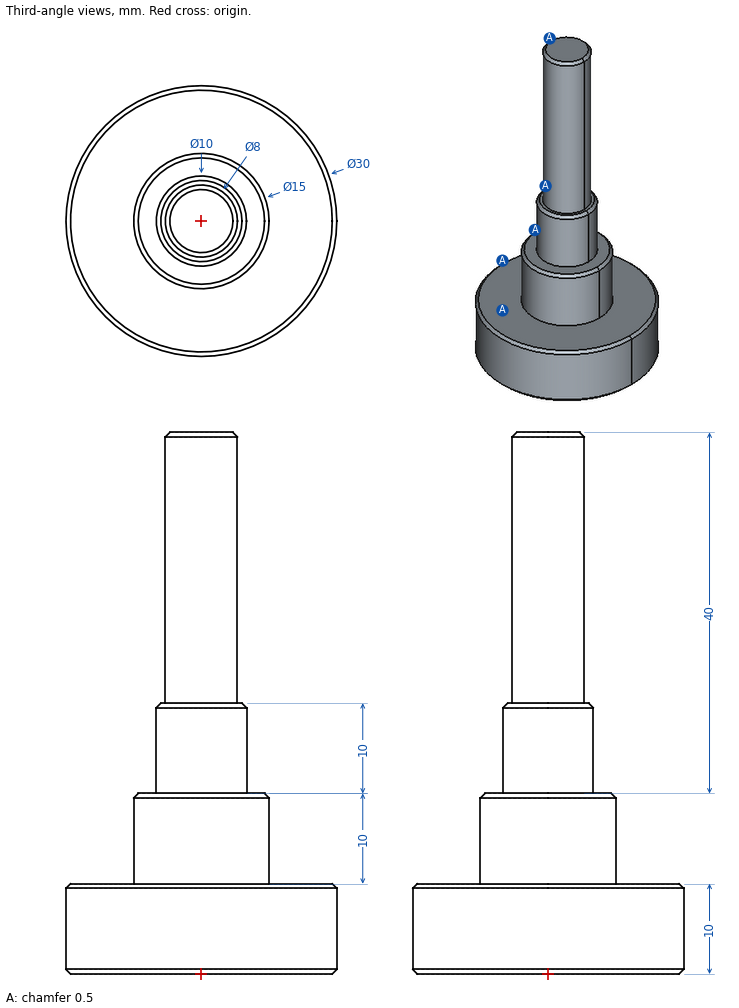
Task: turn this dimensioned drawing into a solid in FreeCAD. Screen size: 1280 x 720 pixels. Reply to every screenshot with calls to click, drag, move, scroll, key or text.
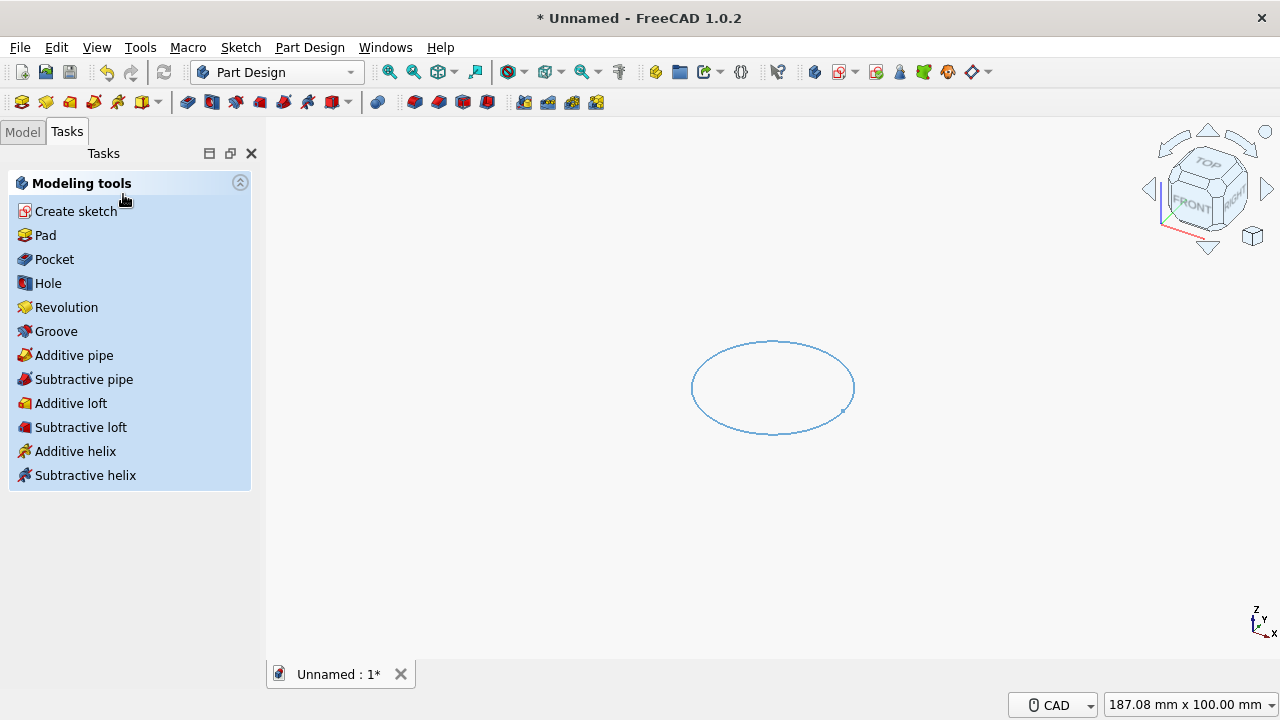
click(22, 102)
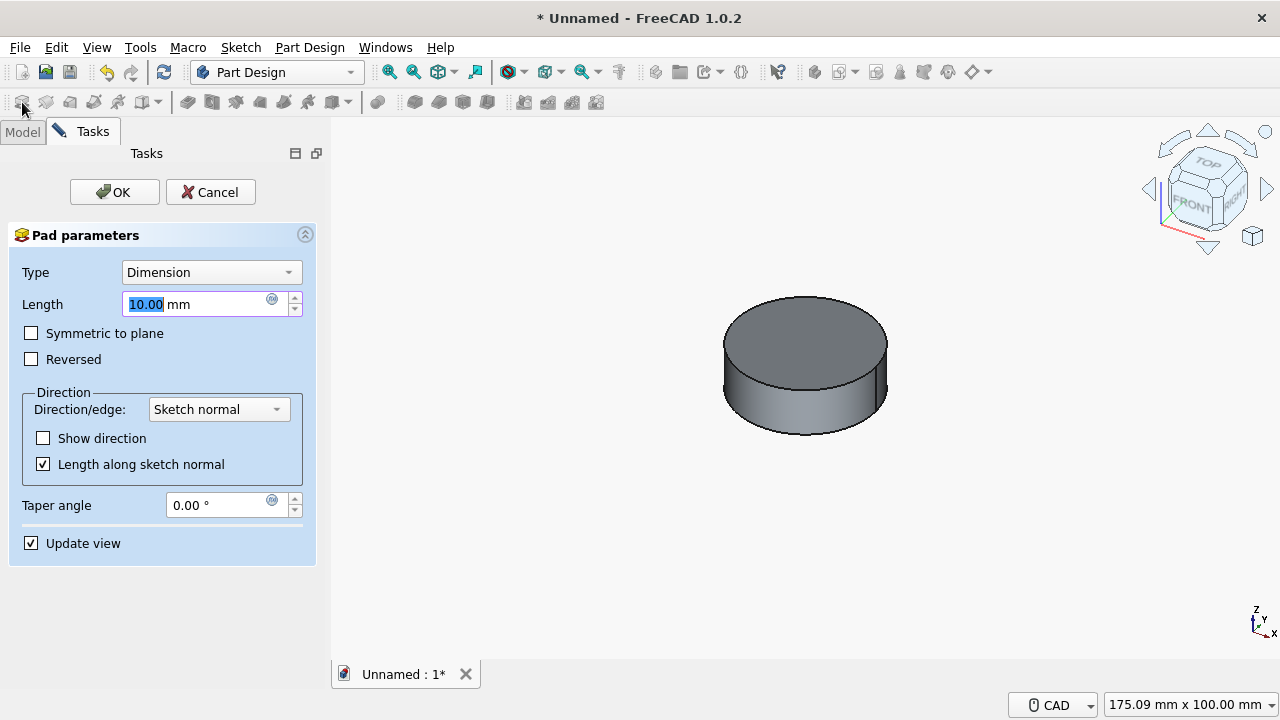
text(10)
key(Tab)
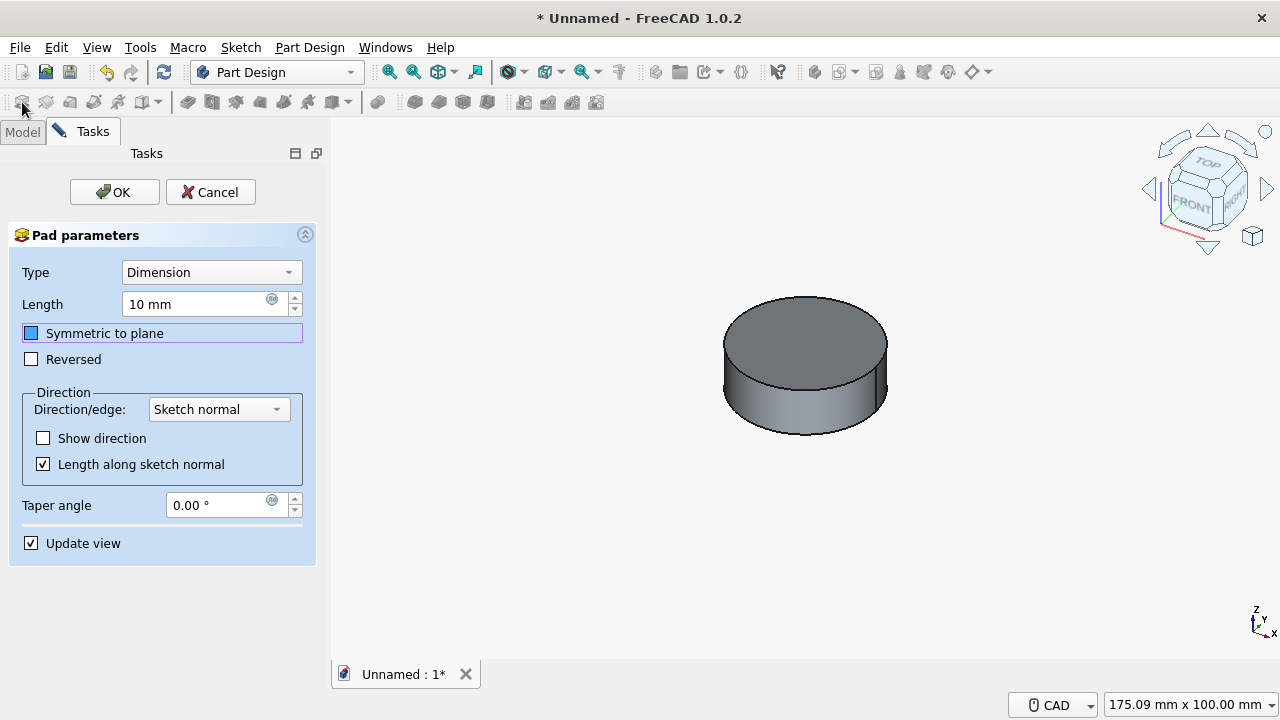
click(115, 192)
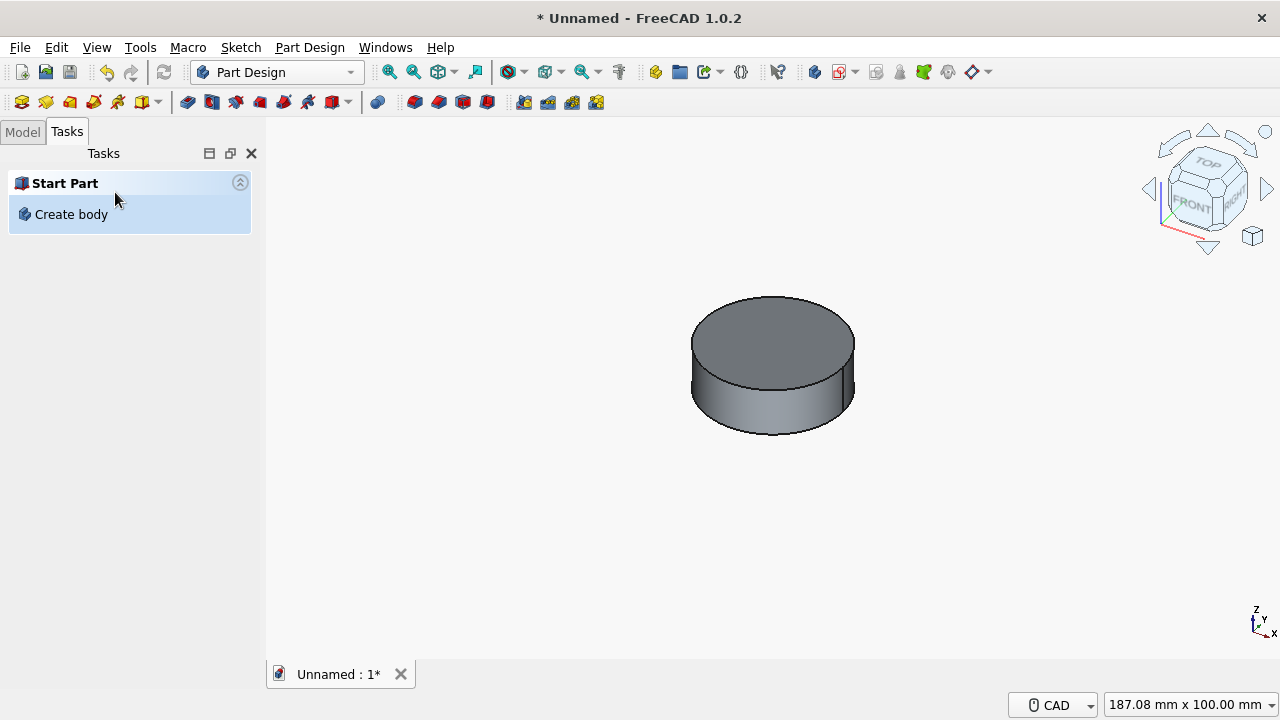
key(v)
key(f)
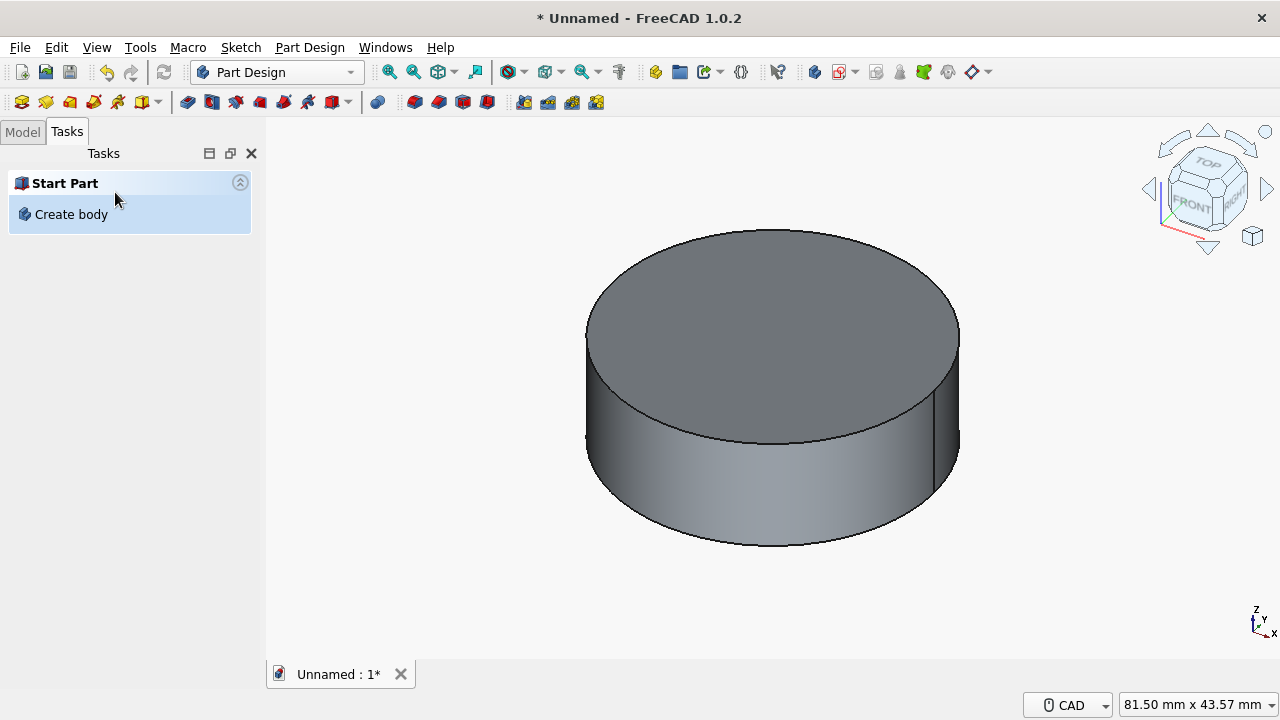
click(773, 336)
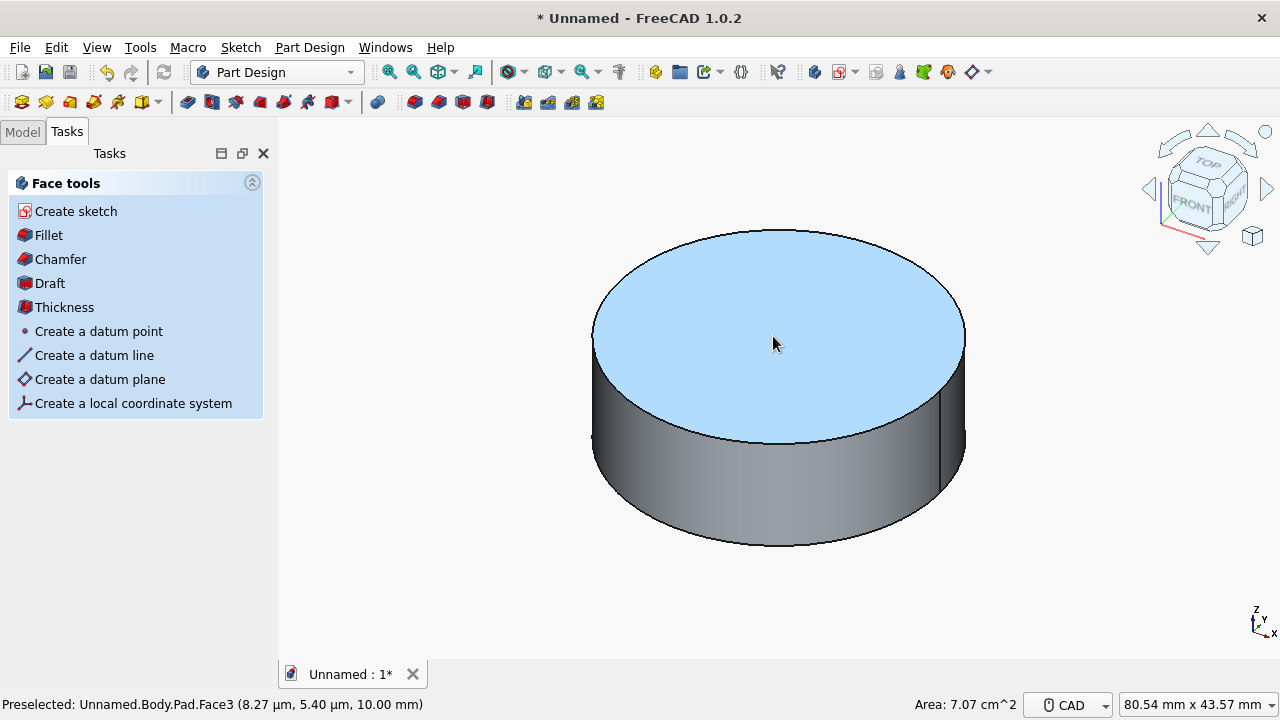
click(840, 72)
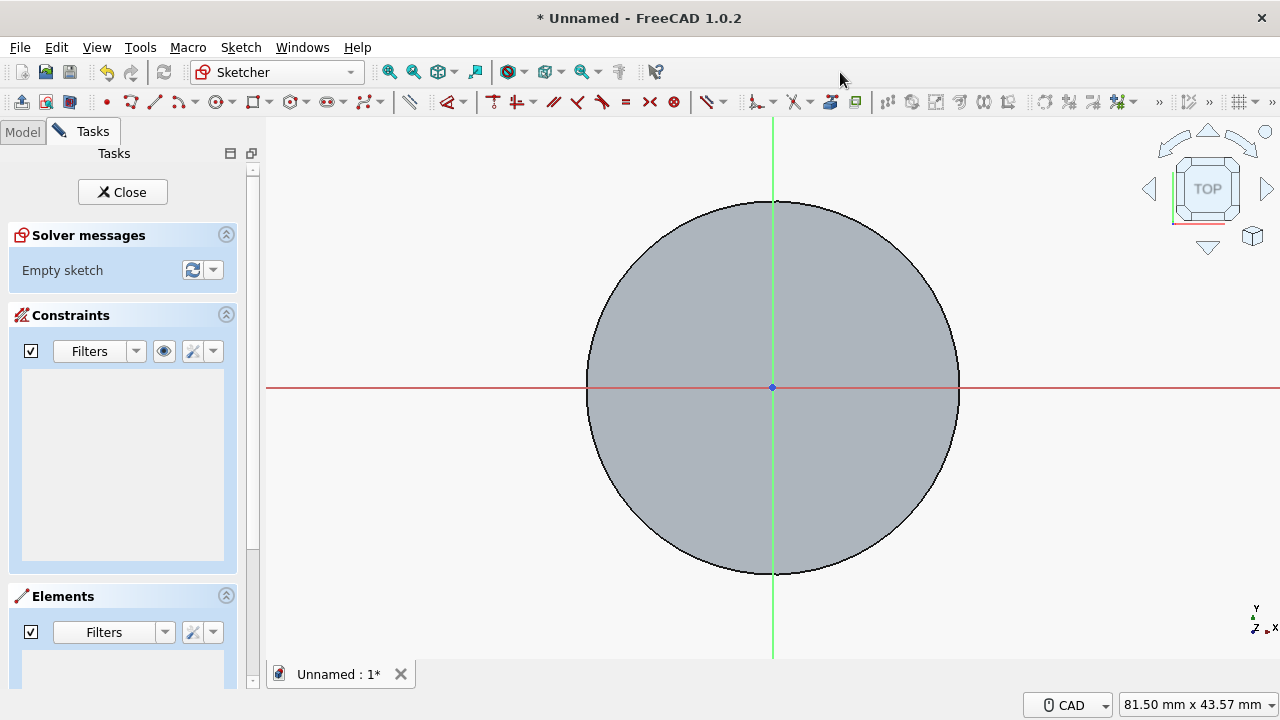
scroll(856, 388, up, 3)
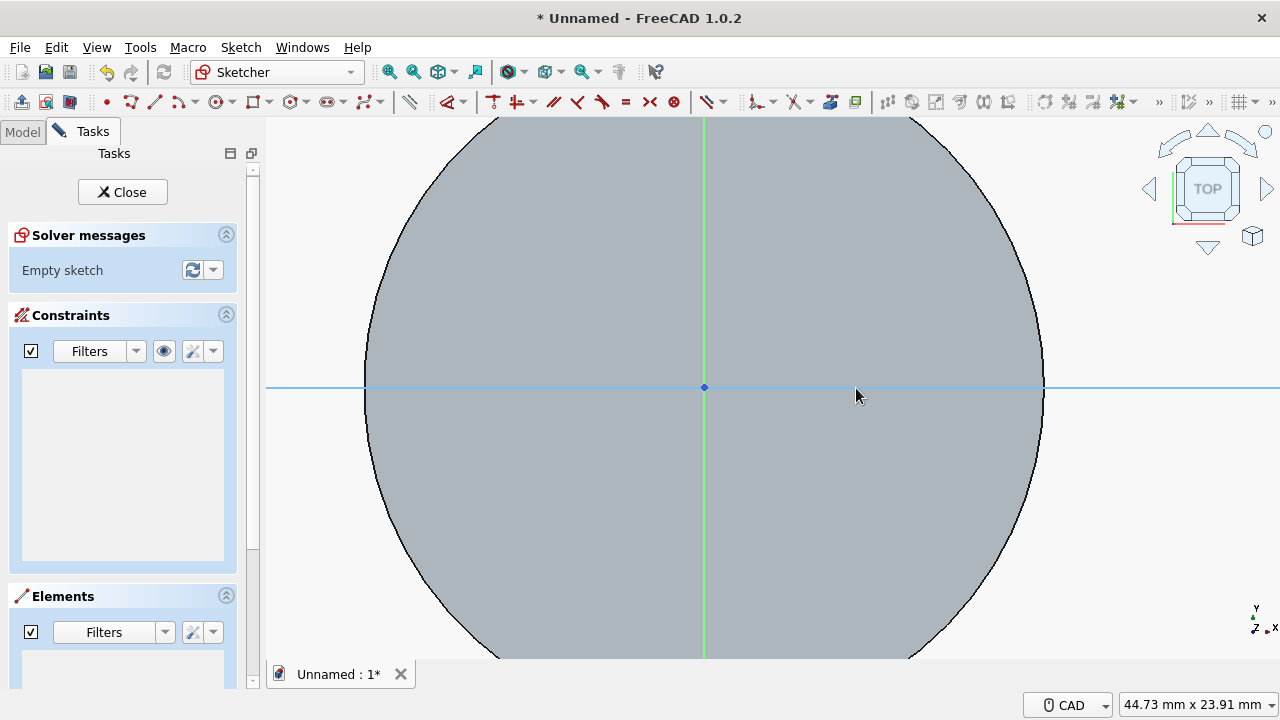
key(g)
key(c)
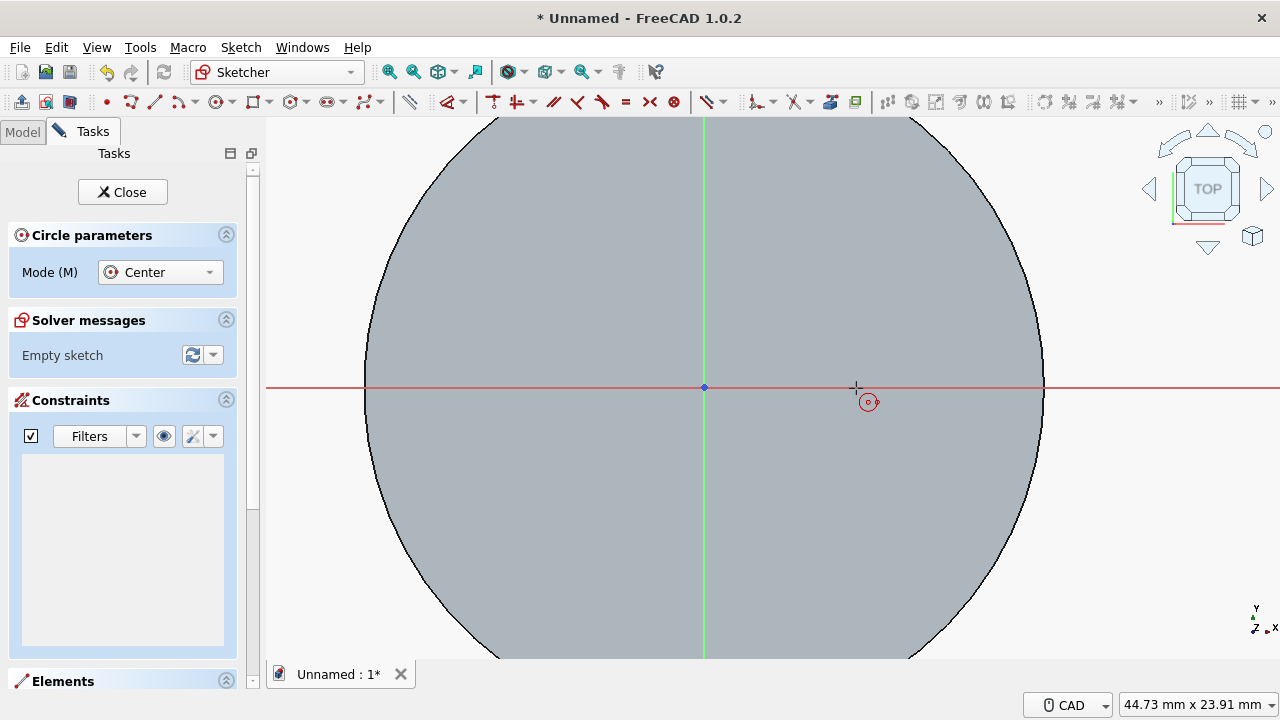
click(704, 388)
click(824, 267)
key(Escape)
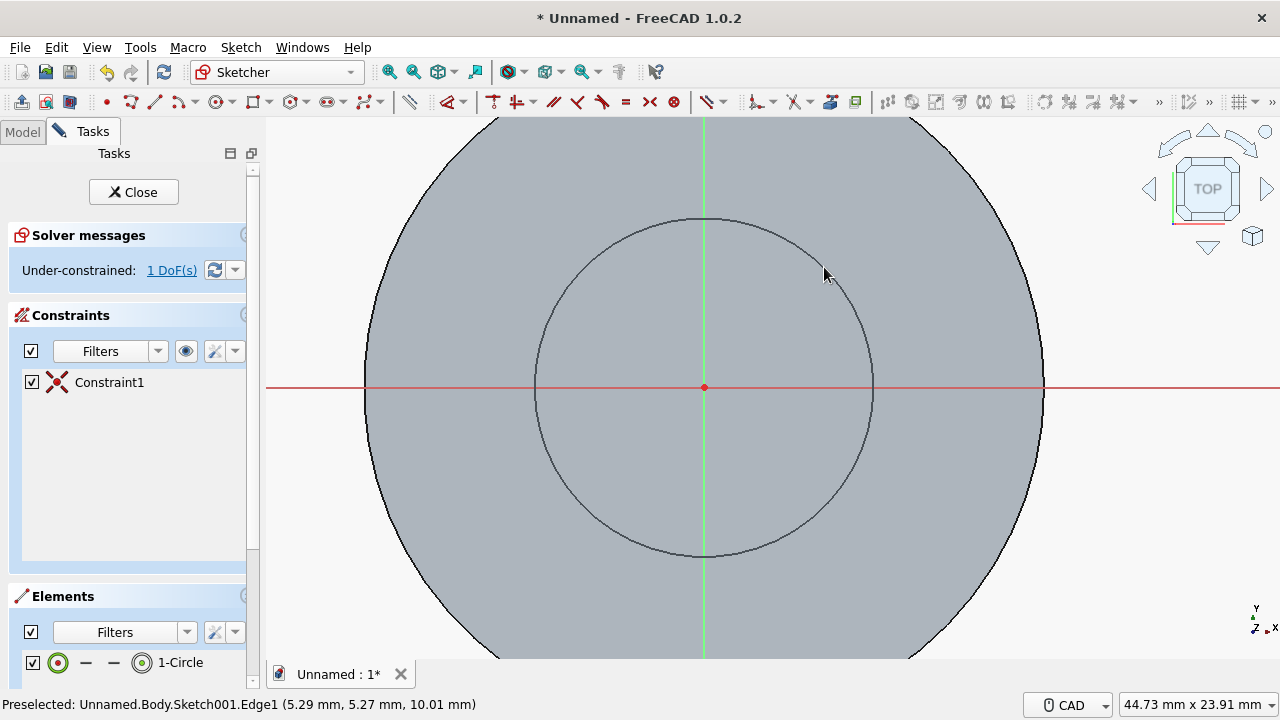
click(823, 267)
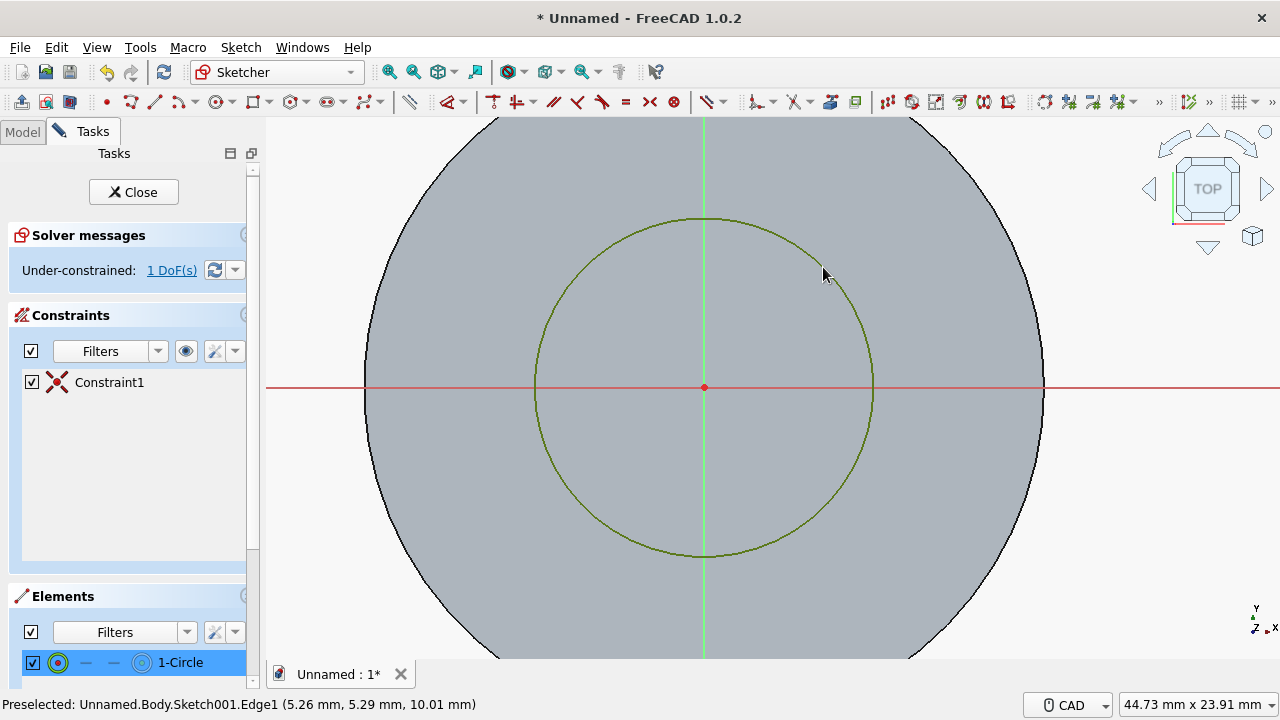
key(k)
key(o)